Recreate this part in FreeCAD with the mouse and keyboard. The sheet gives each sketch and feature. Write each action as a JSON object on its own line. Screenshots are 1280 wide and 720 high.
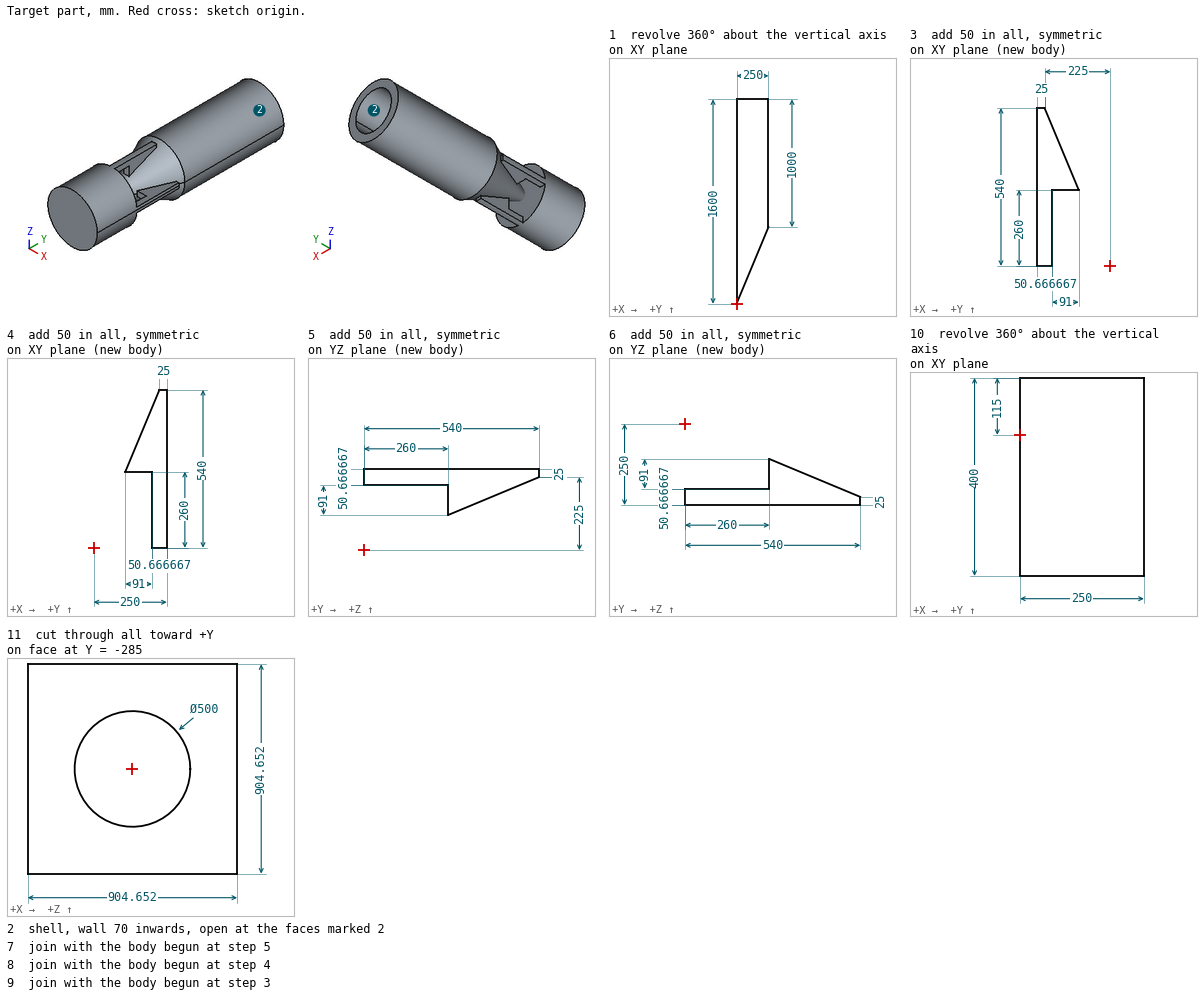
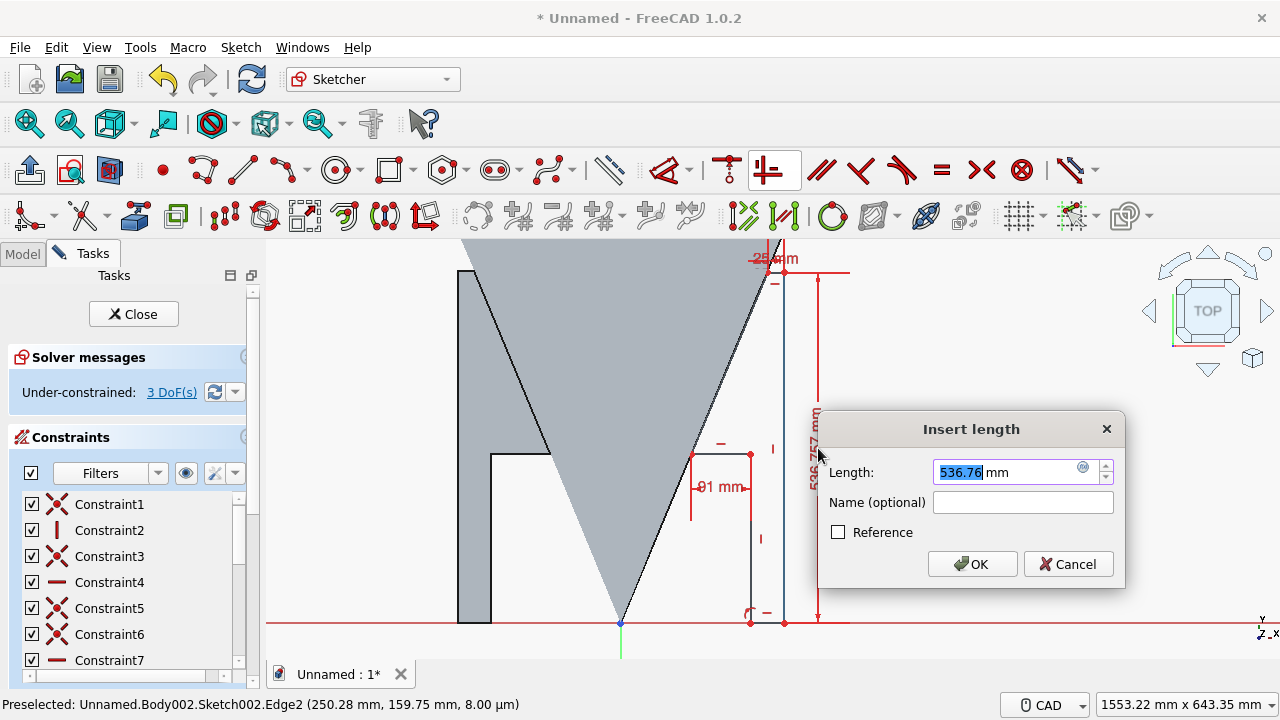
{"action": "type", "text": "540"}
{"action": "key", "text": "Return"}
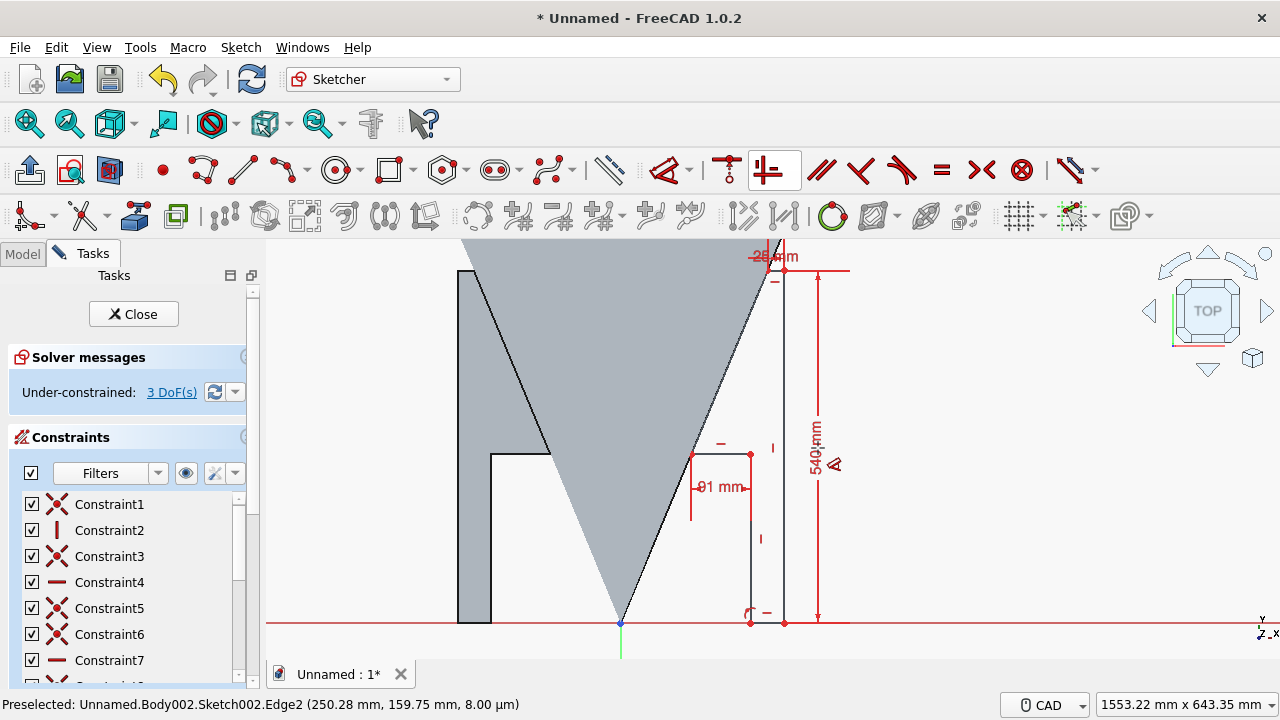
{"action": "left_click", "coordinate": [751, 505]}
{"action": "left_click", "coordinate": [717, 539]}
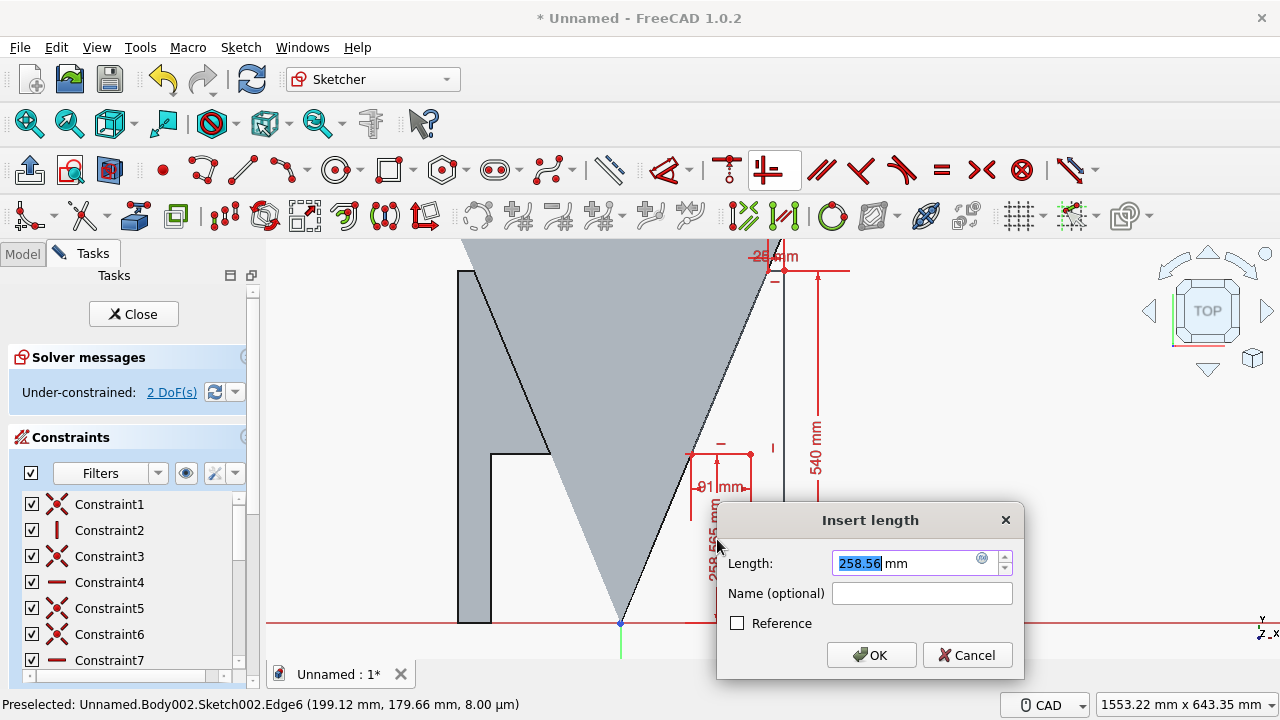
{"action": "type", "text": "260"}
{"action": "key", "text": "Return"}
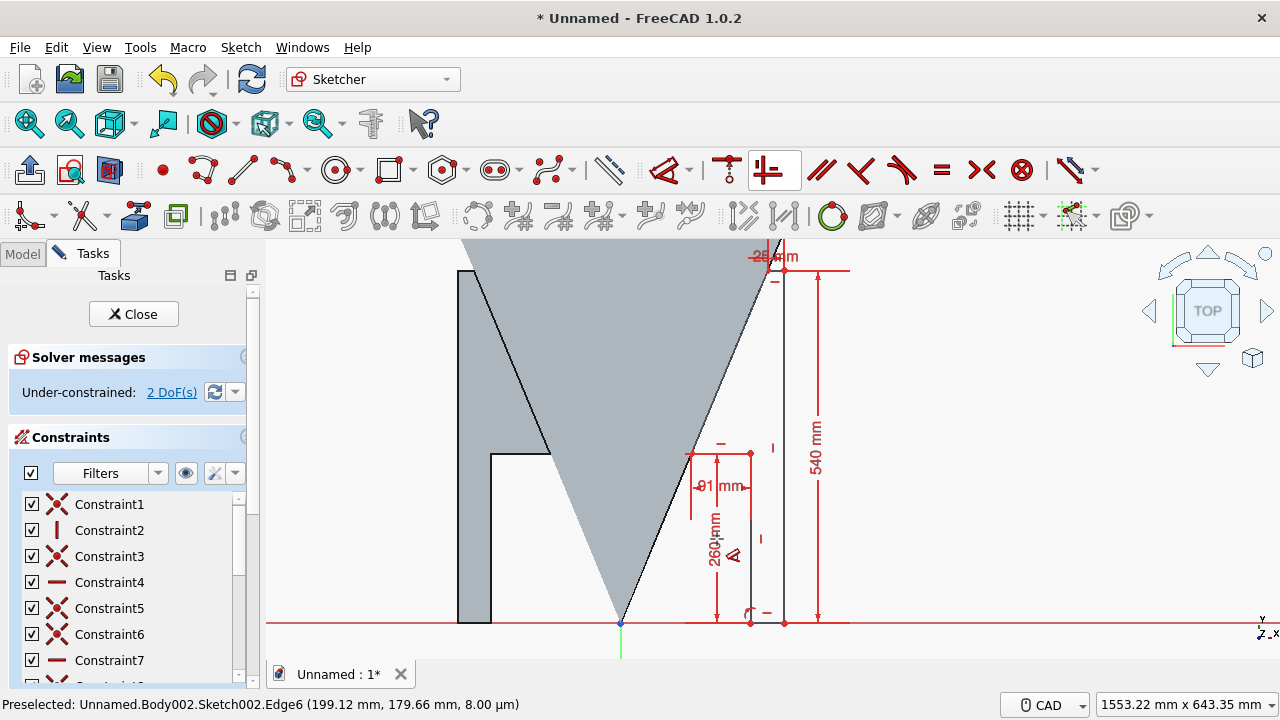
{"action": "left_click", "coordinate": [784, 623]}
{"action": "left_click", "coordinate": [702, 589]}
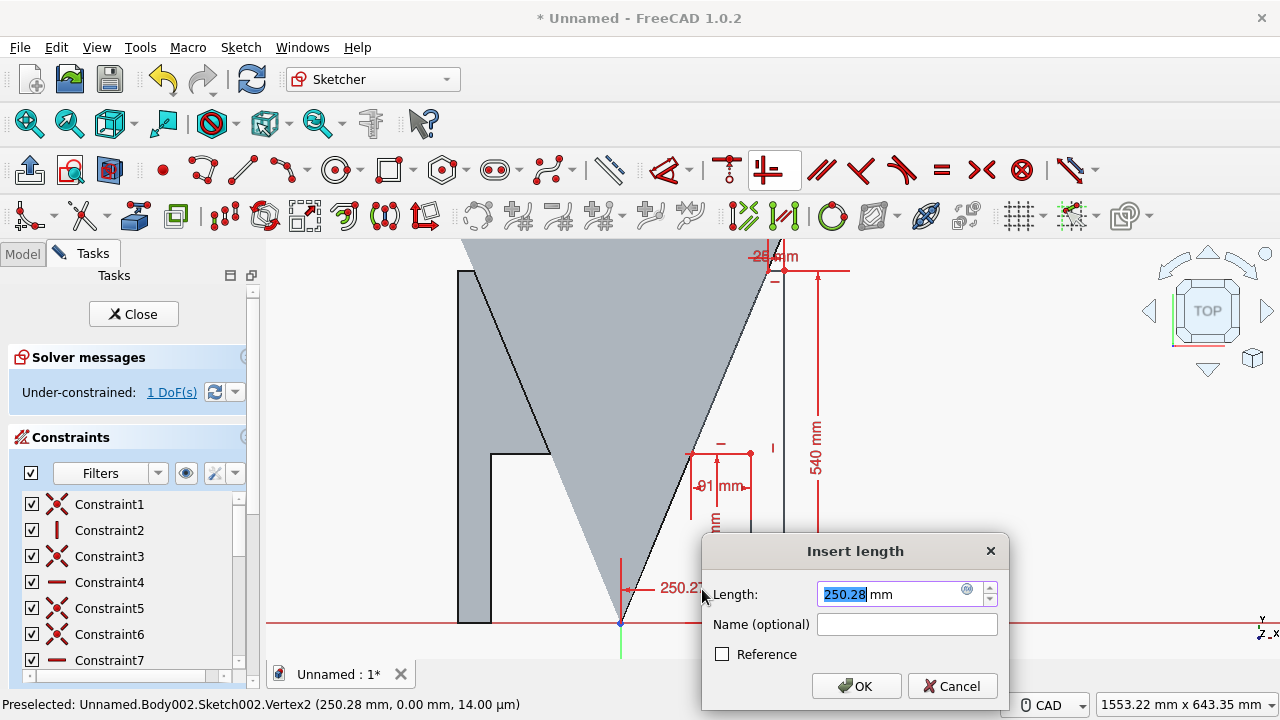
{"action": "type", "text": "250"}
{"action": "key", "text": "Return"}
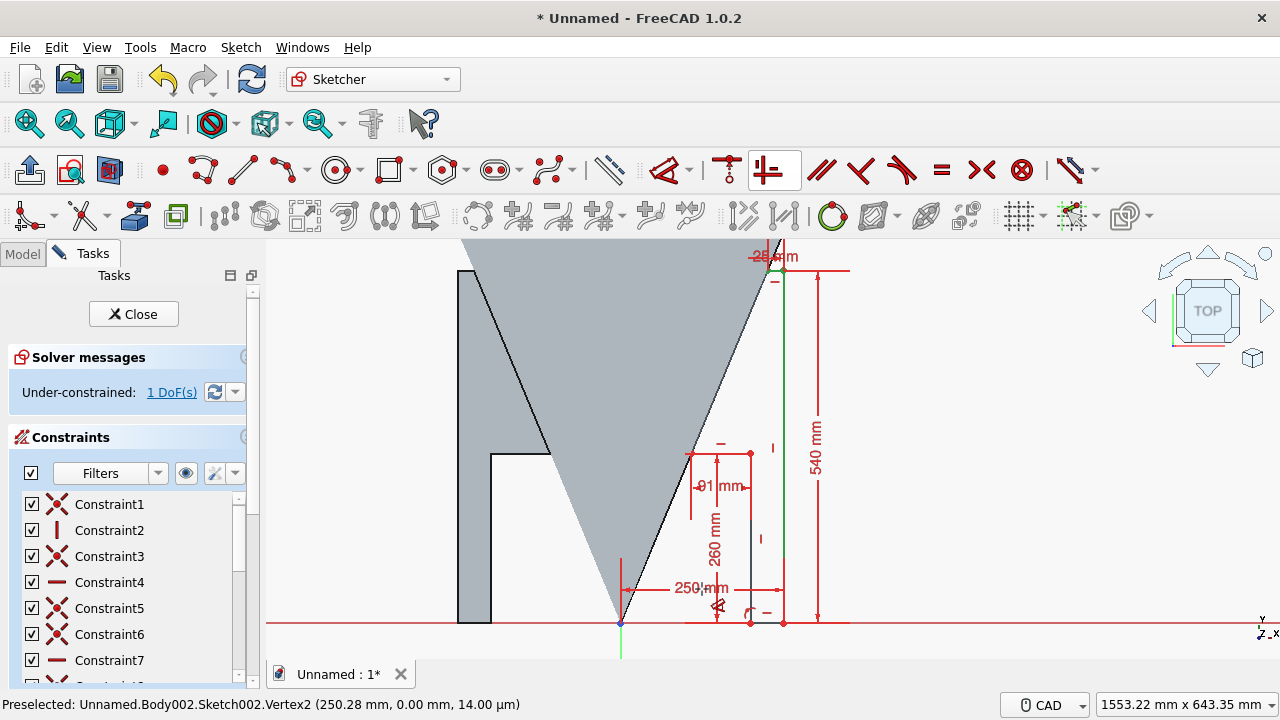
{"action": "scroll", "coordinate": [761, 623], "scroll_direction": "up", "scroll_amount": 2}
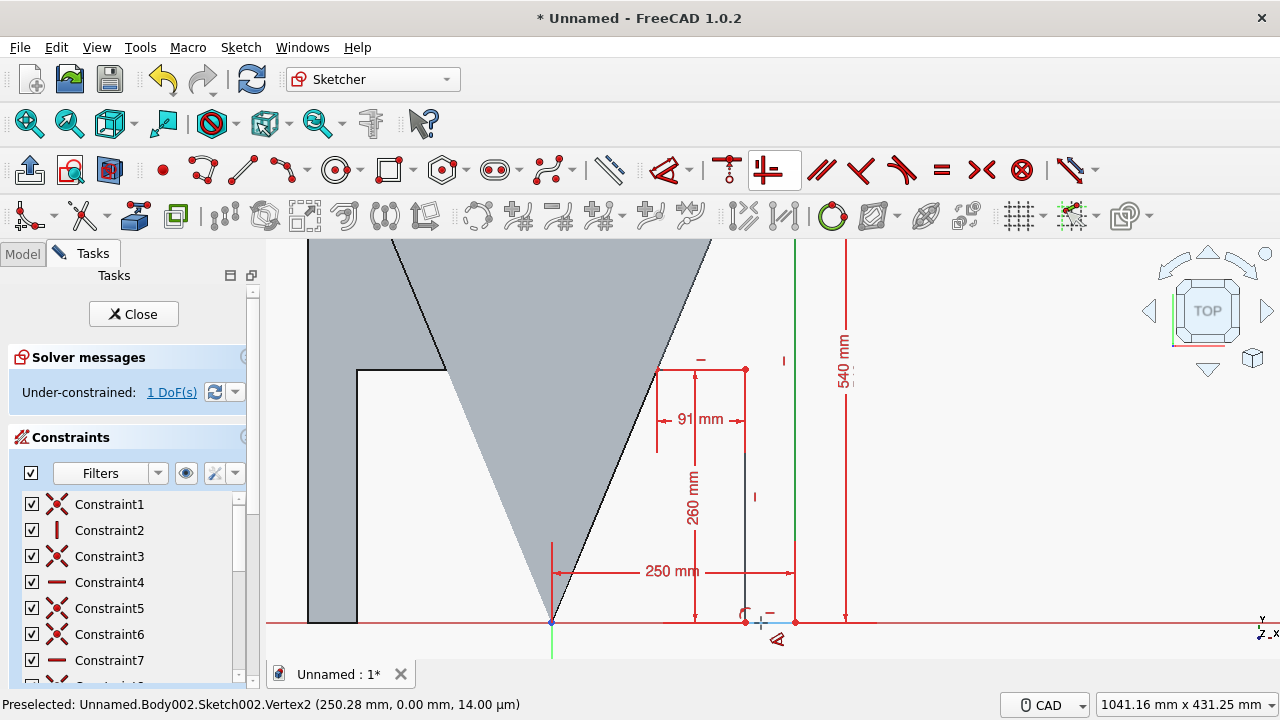
{"action": "left_click", "coordinate": [760, 623]}
{"action": "left_click", "coordinate": [770, 589]}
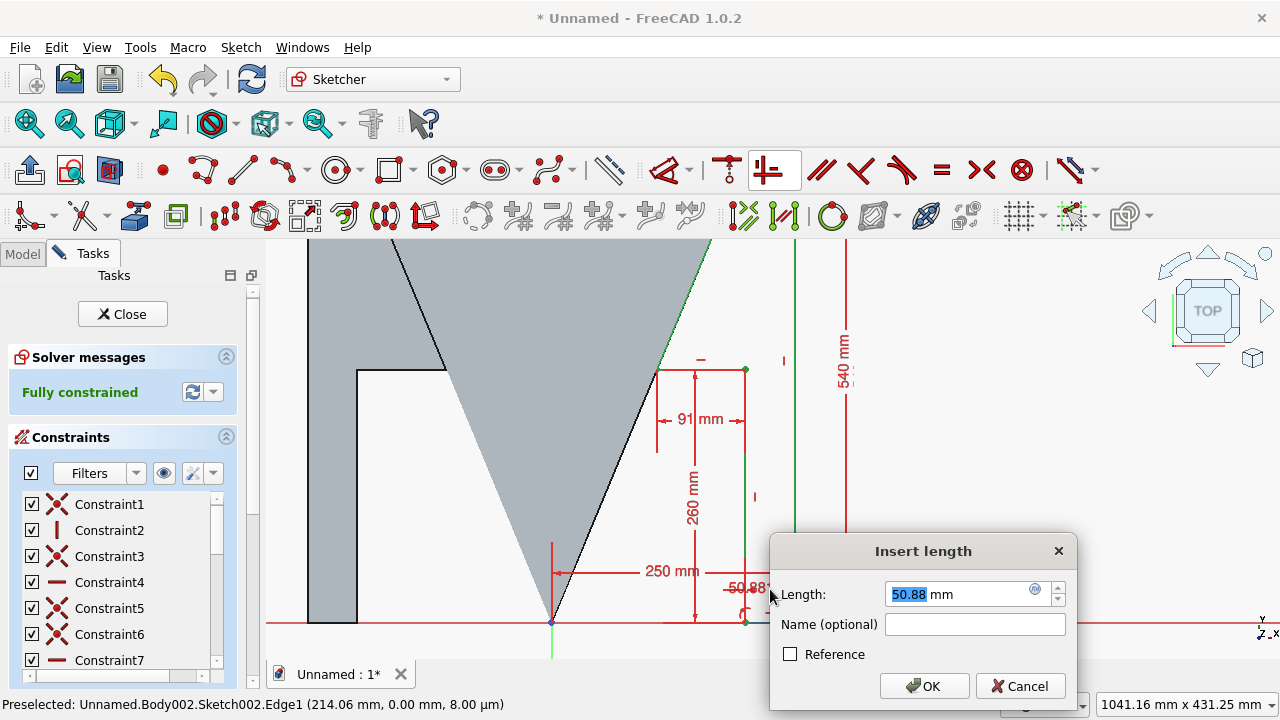
{"action": "type", "text": "50.666667"}
{"action": "key", "text": "Return"}
{"action": "key", "text": "Escape"}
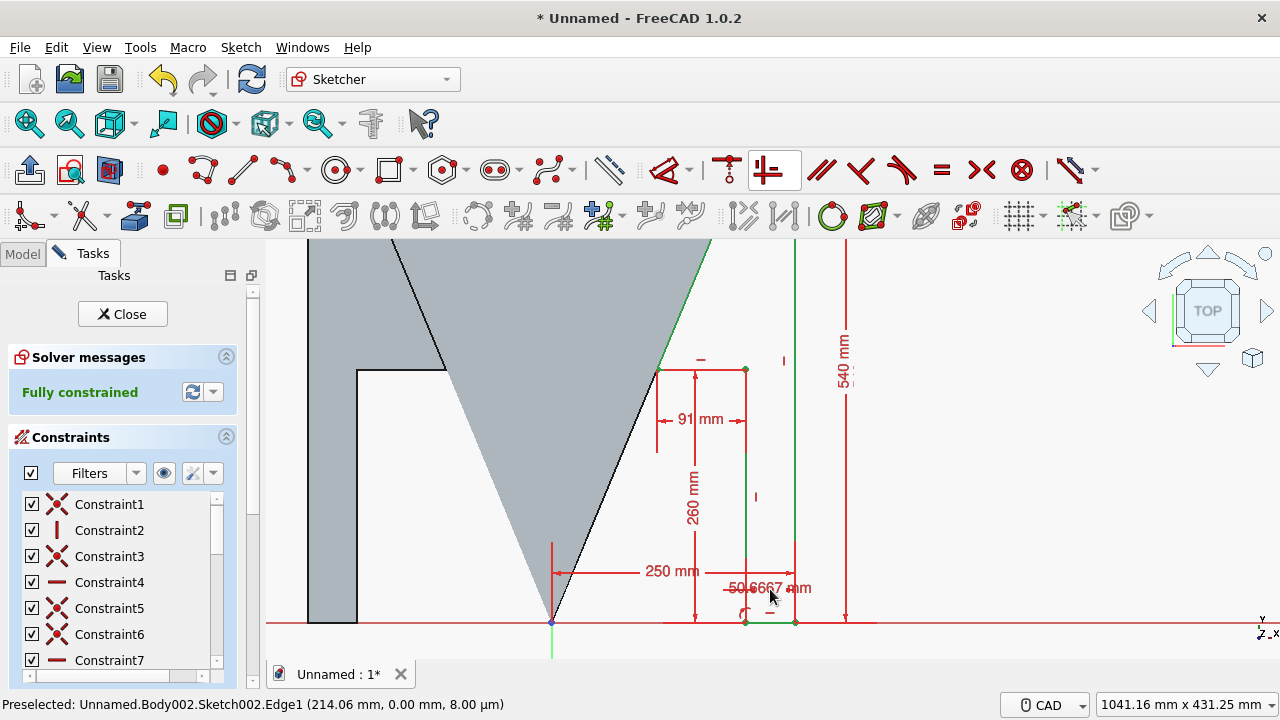
{"action": "left_click", "coordinate": [123, 314]}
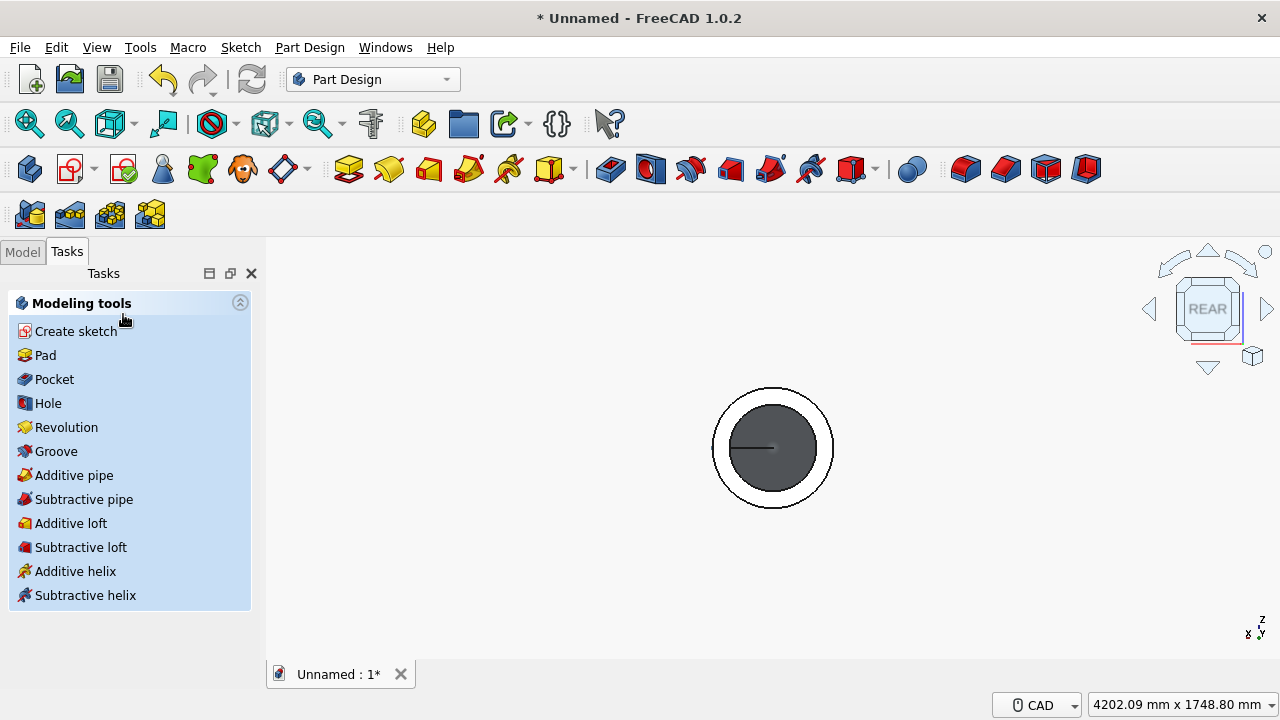
{"action": "left_click", "coordinate": [350, 170]}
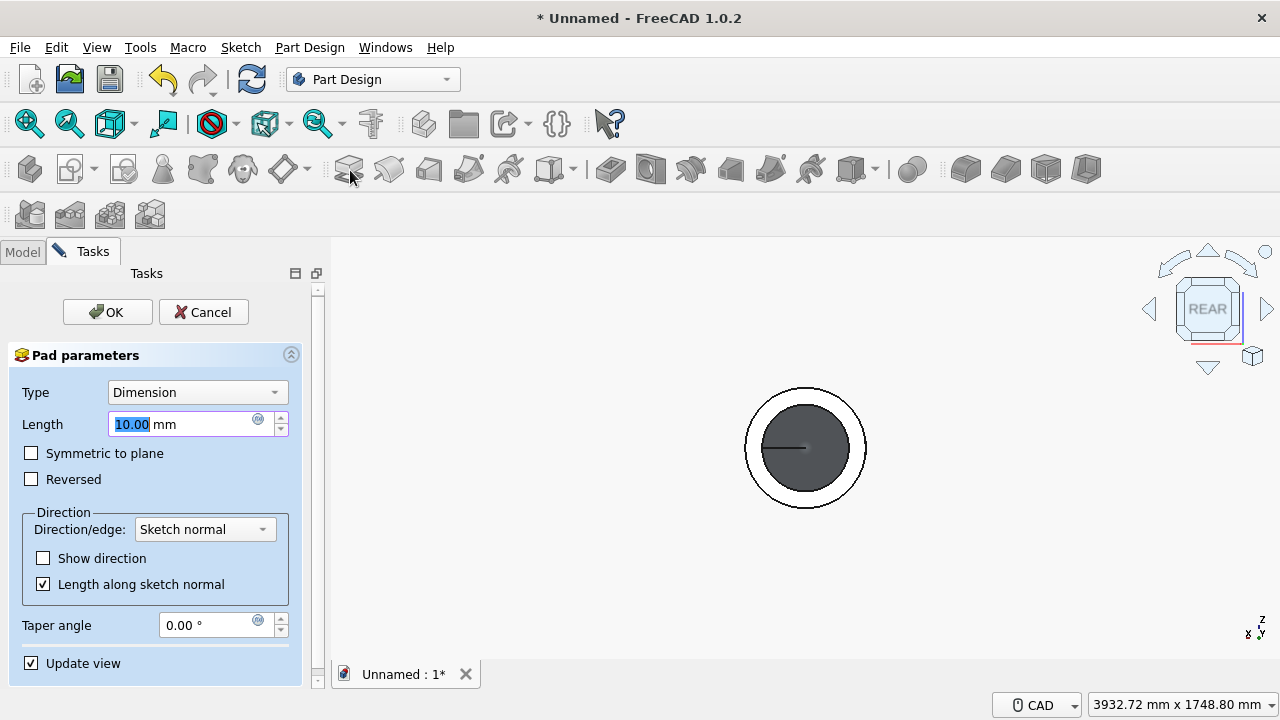
{"action": "type", "text": "50"}
{"action": "key", "text": "Tab"}